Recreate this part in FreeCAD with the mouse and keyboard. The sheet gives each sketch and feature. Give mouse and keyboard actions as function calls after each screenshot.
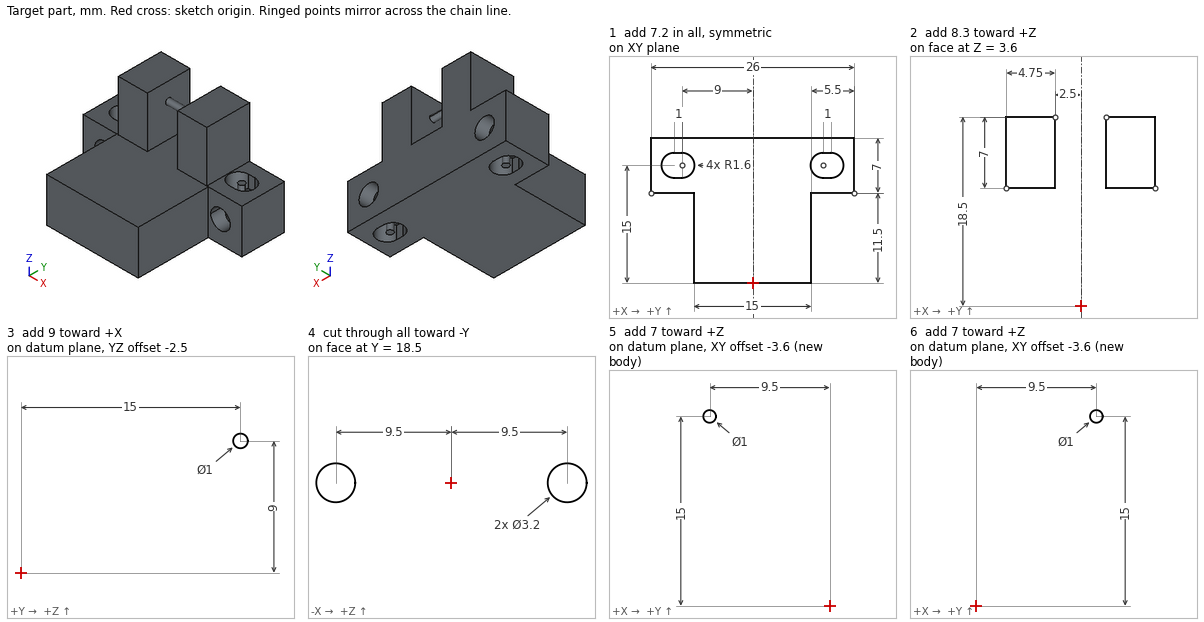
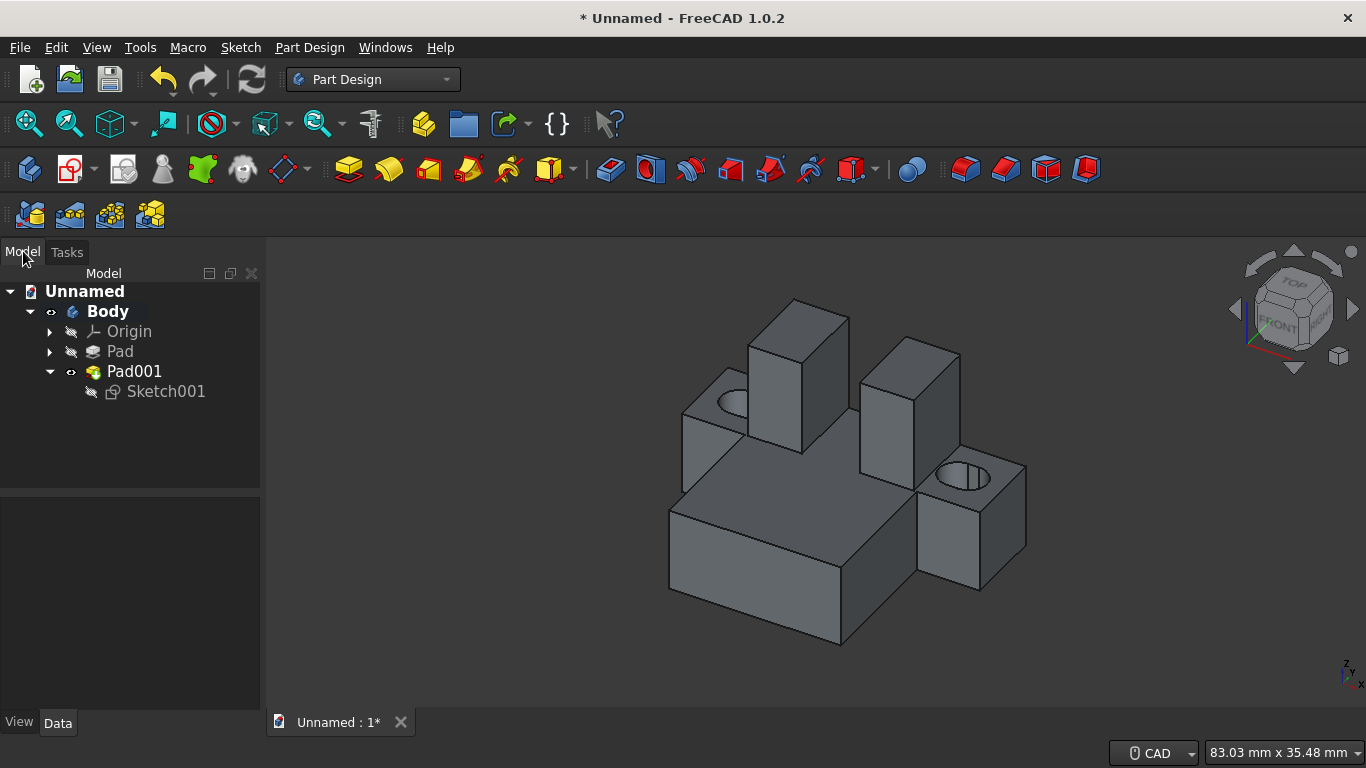
click(50, 332)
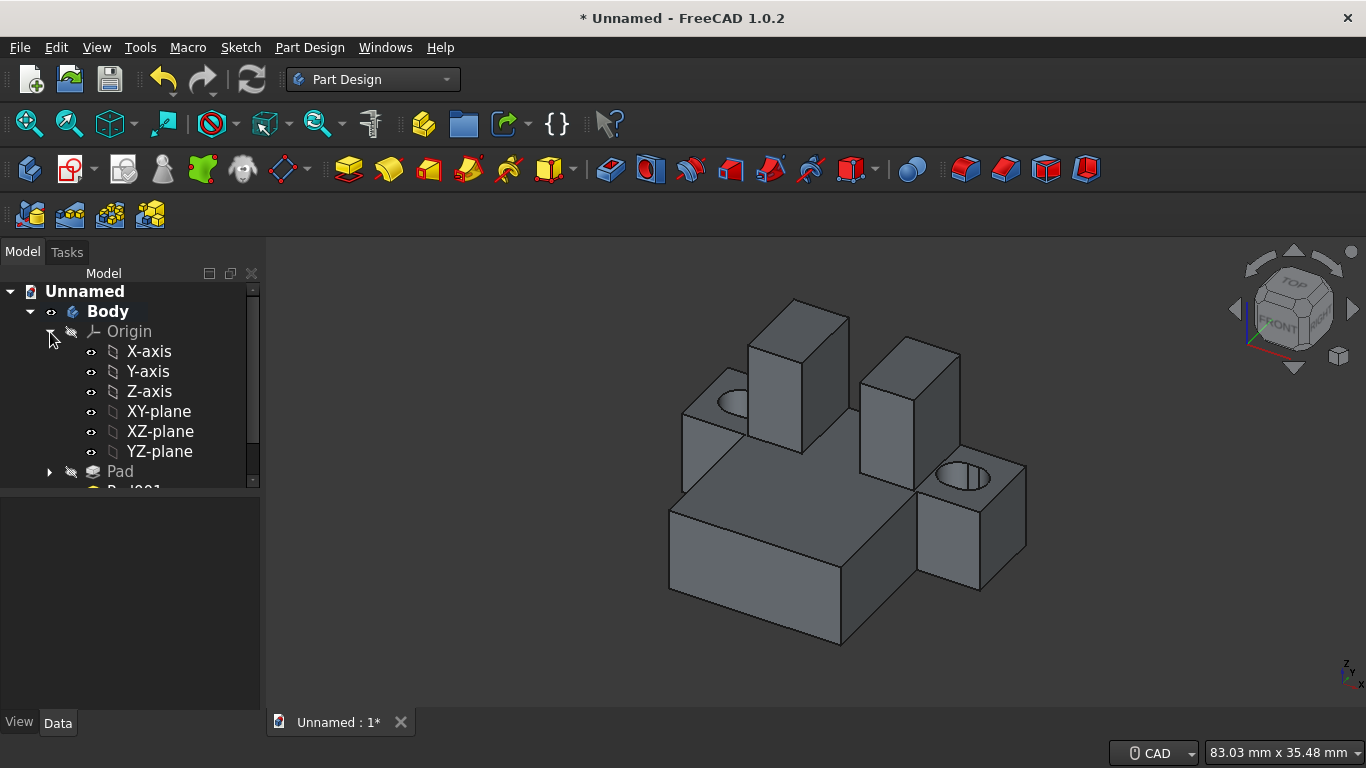
click(136, 452)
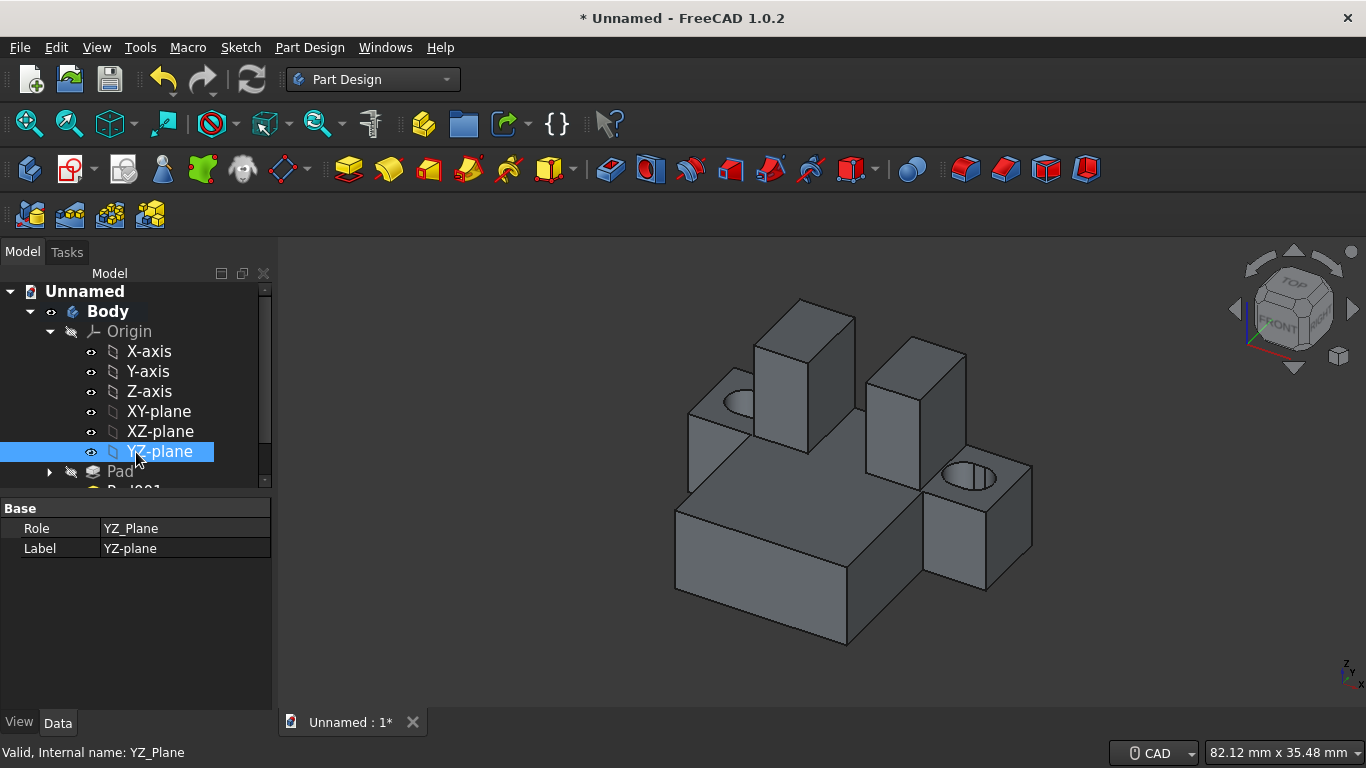
click(284, 170)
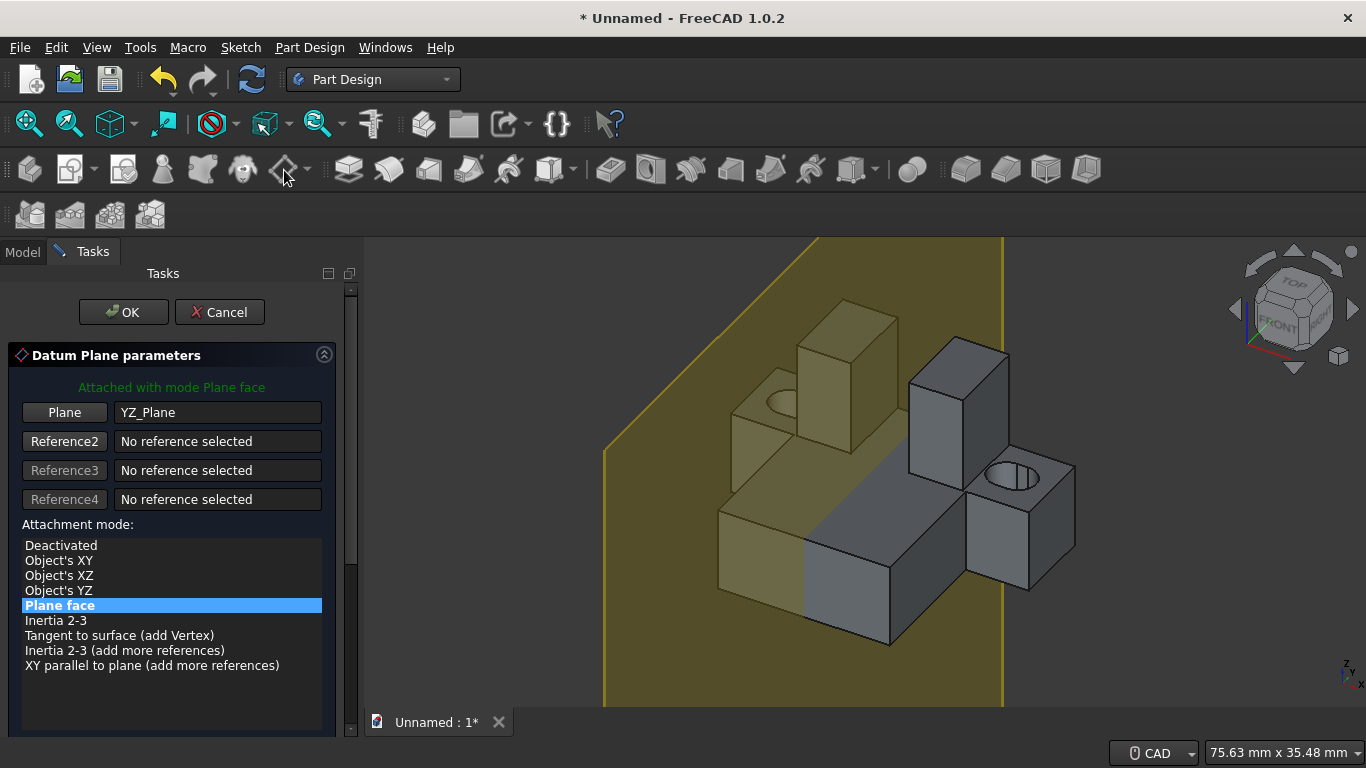
scroll(351, 510, down, 3)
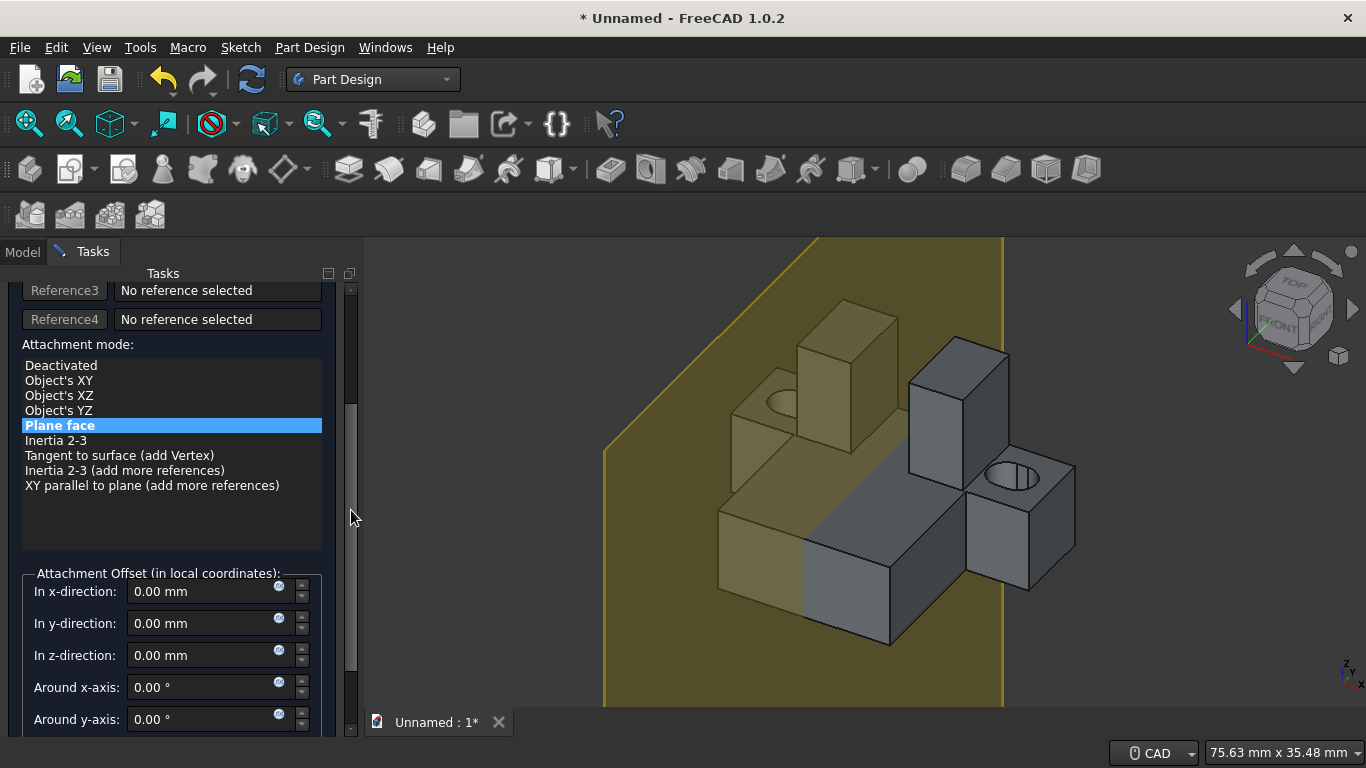
triple_click(210, 655)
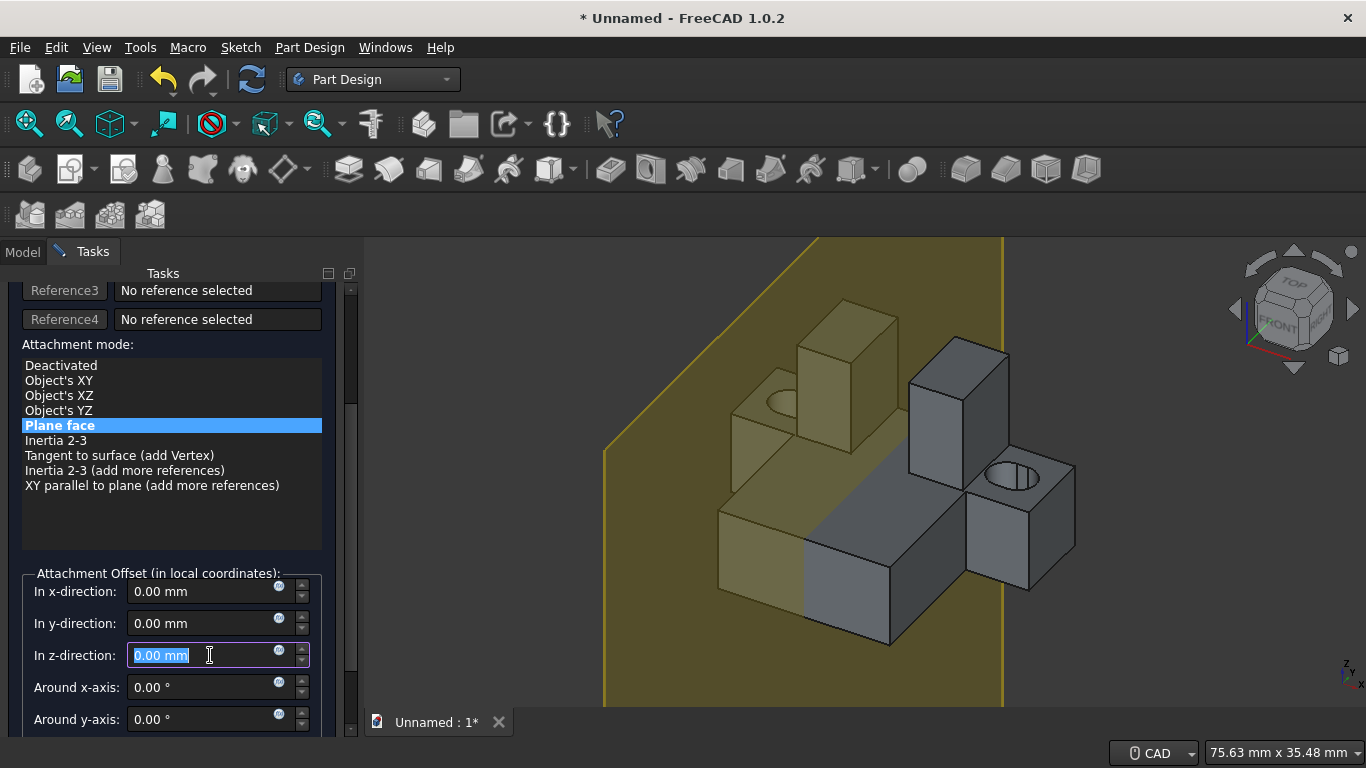
text(-2.5)
key(Tab)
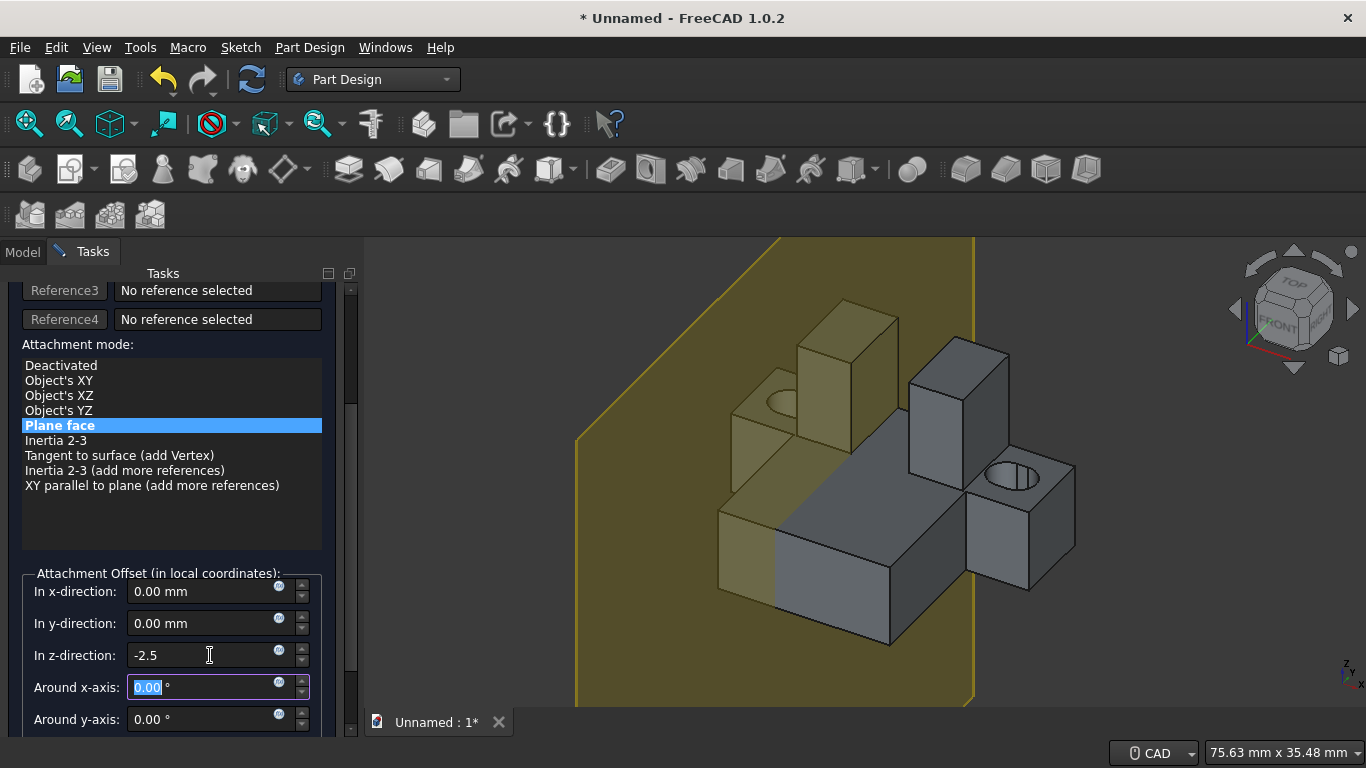
scroll(351, 510, up, 4)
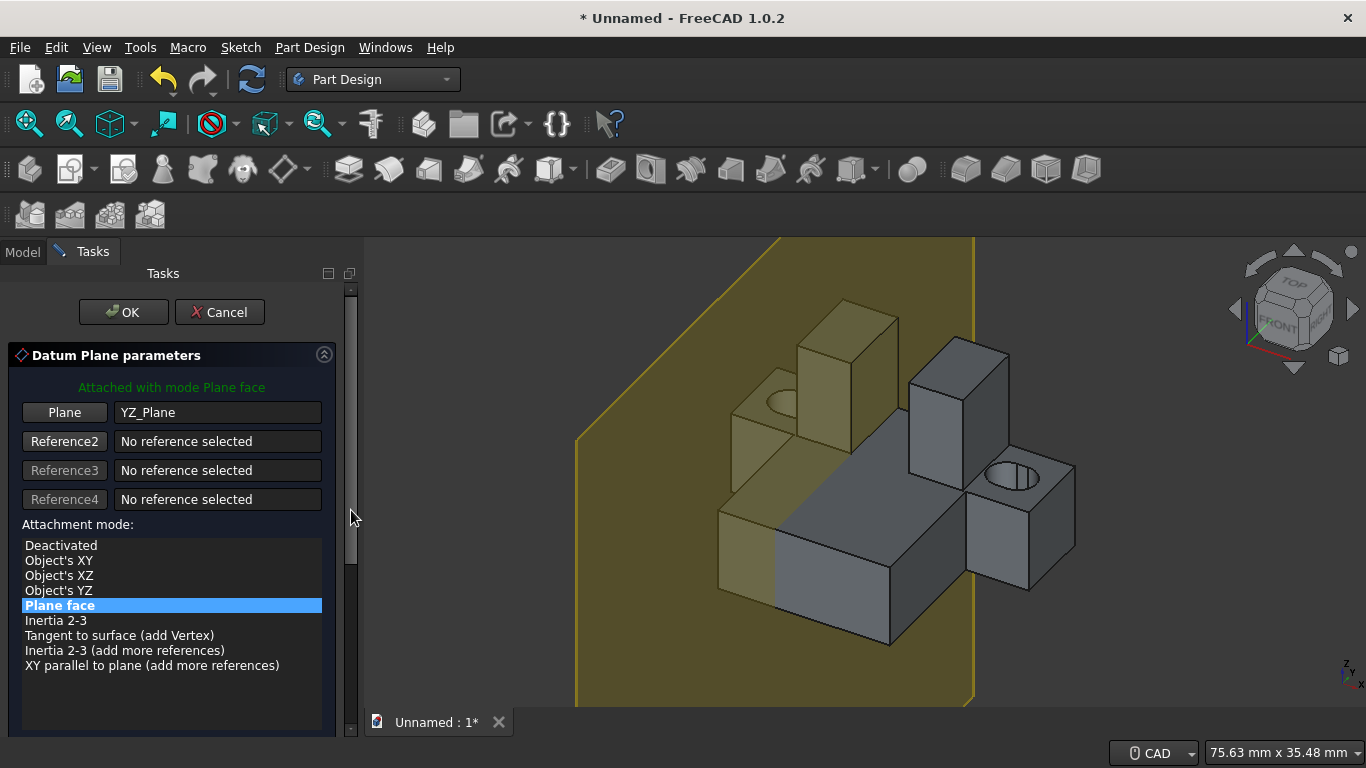
click(124, 312)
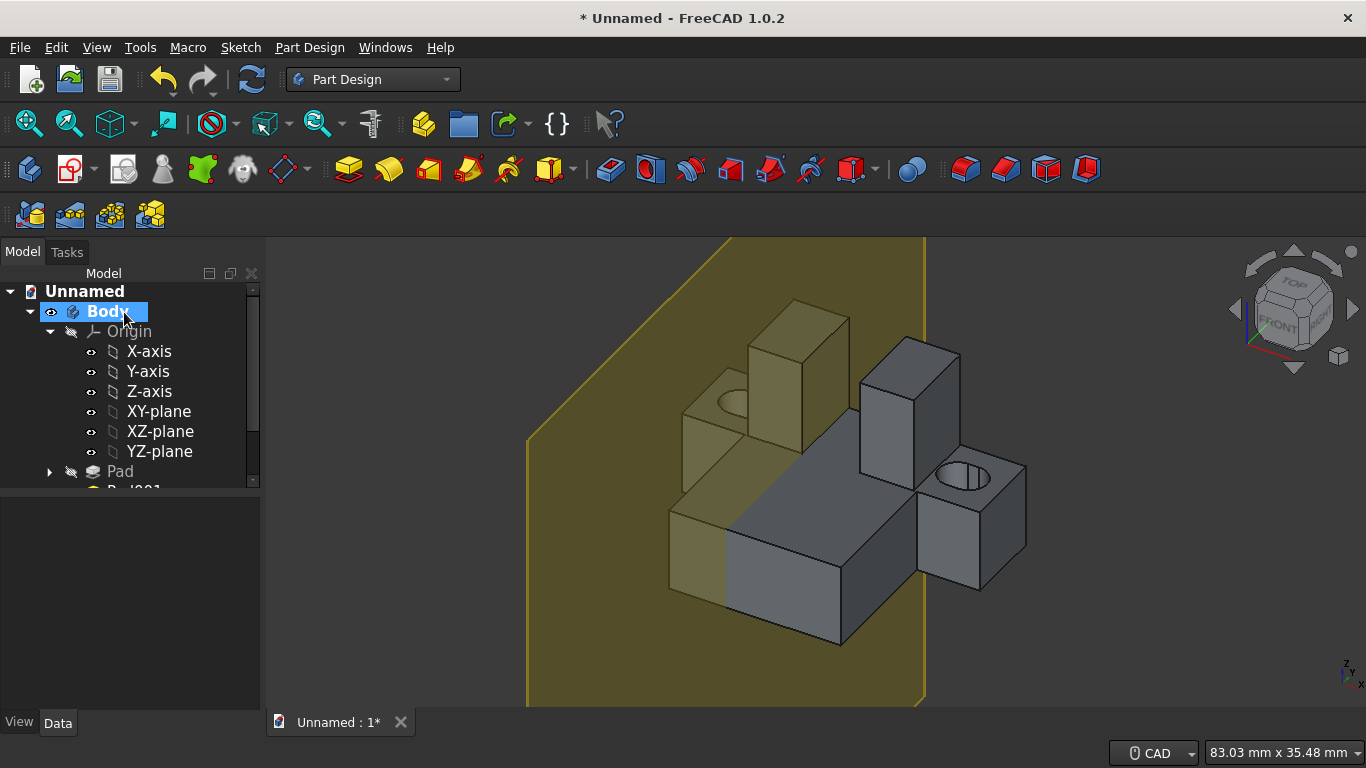
scroll(100, 387, down, 3)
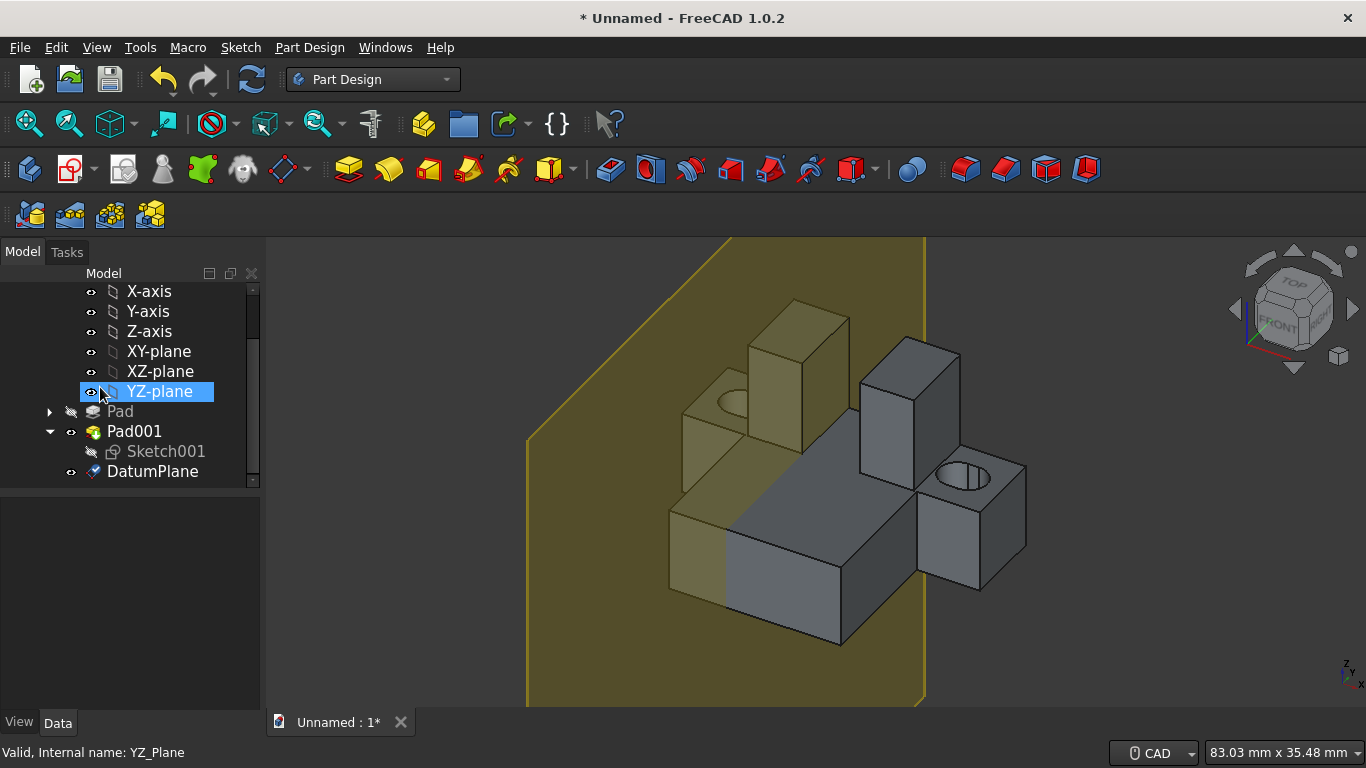
click(116, 472)